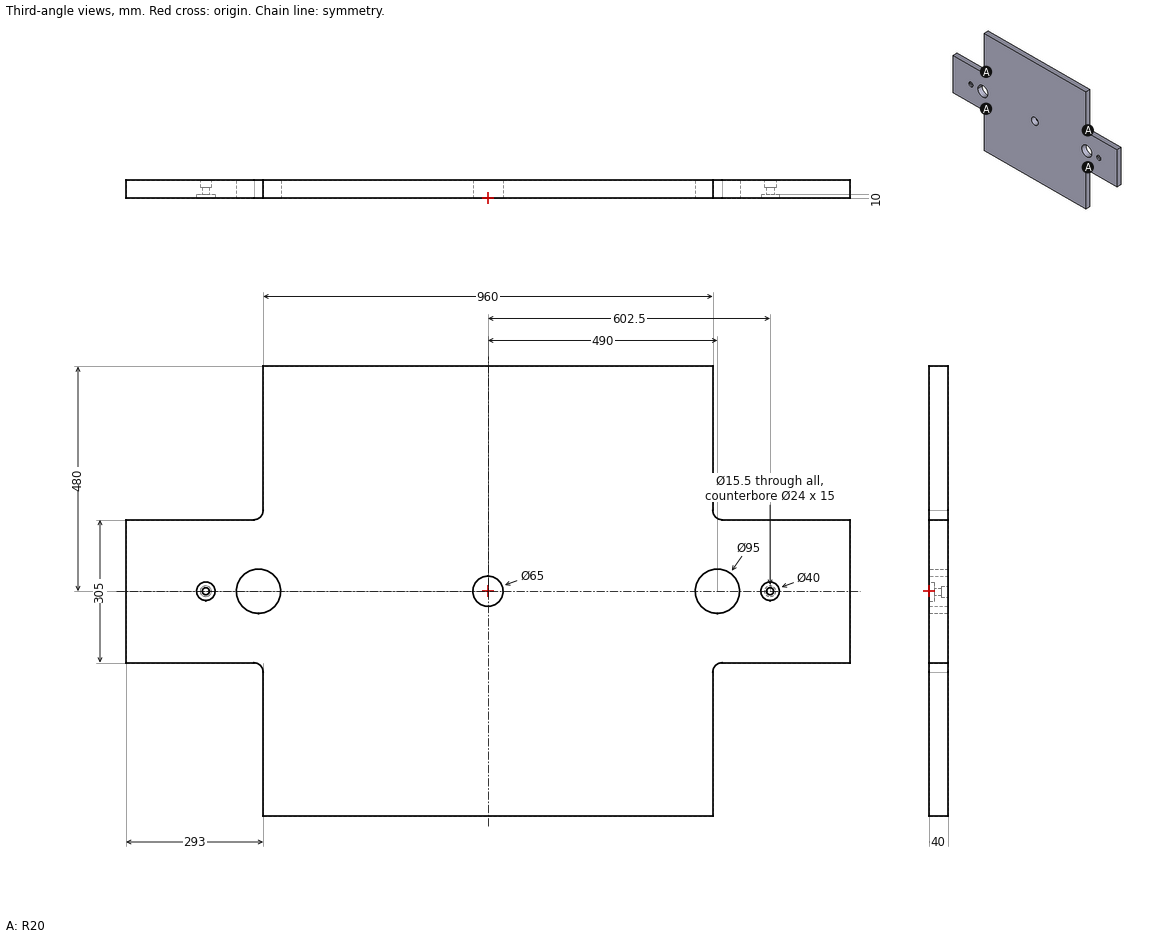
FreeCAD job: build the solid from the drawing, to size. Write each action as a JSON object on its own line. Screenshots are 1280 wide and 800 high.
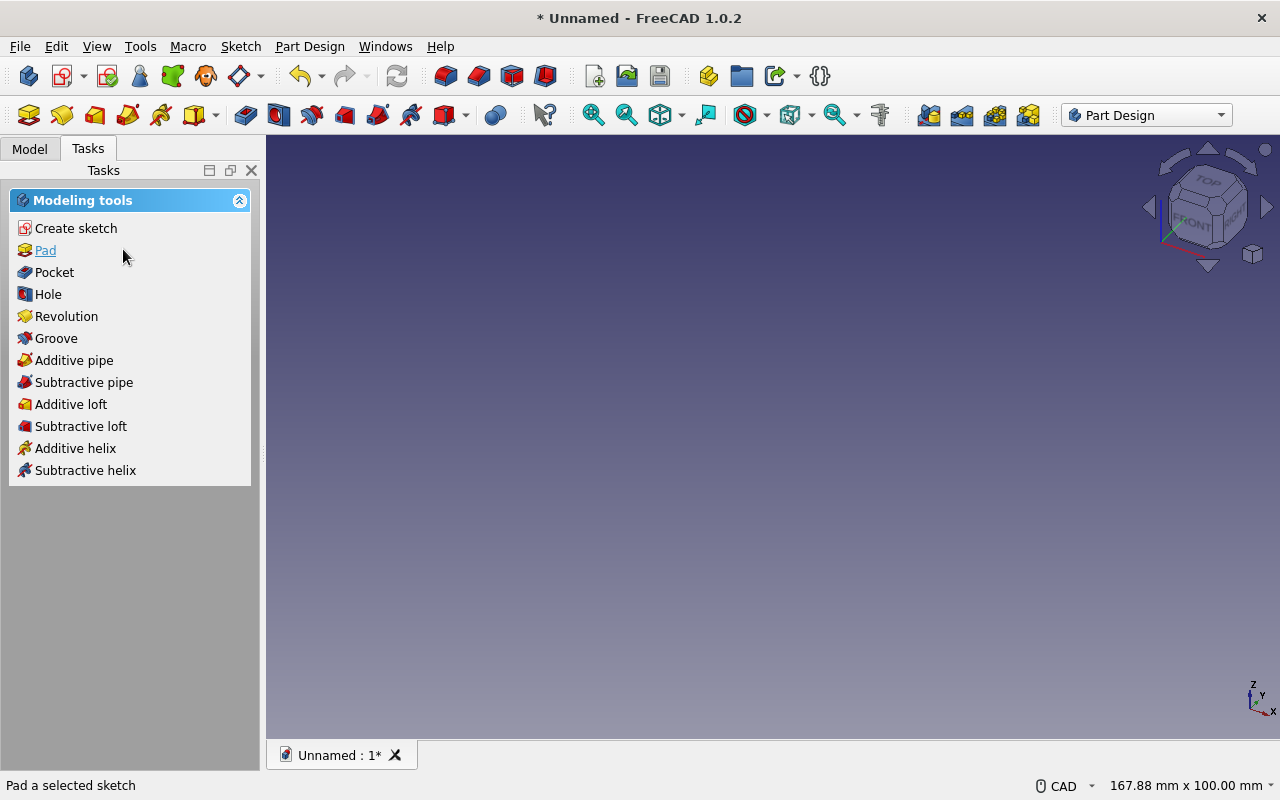
{"action": "left_click", "coordinate": [29, 116]}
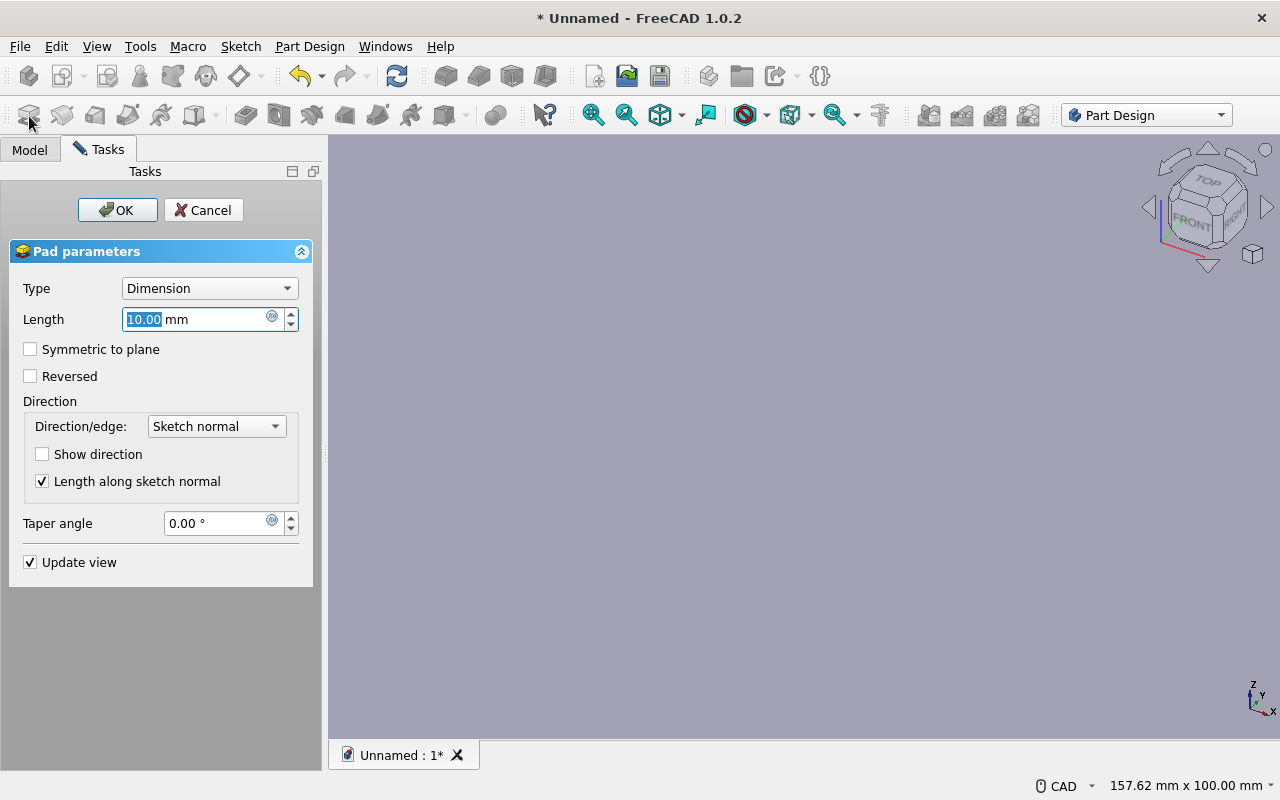
{"action": "type", "text": "40"}
{"action": "key", "text": "Tab"}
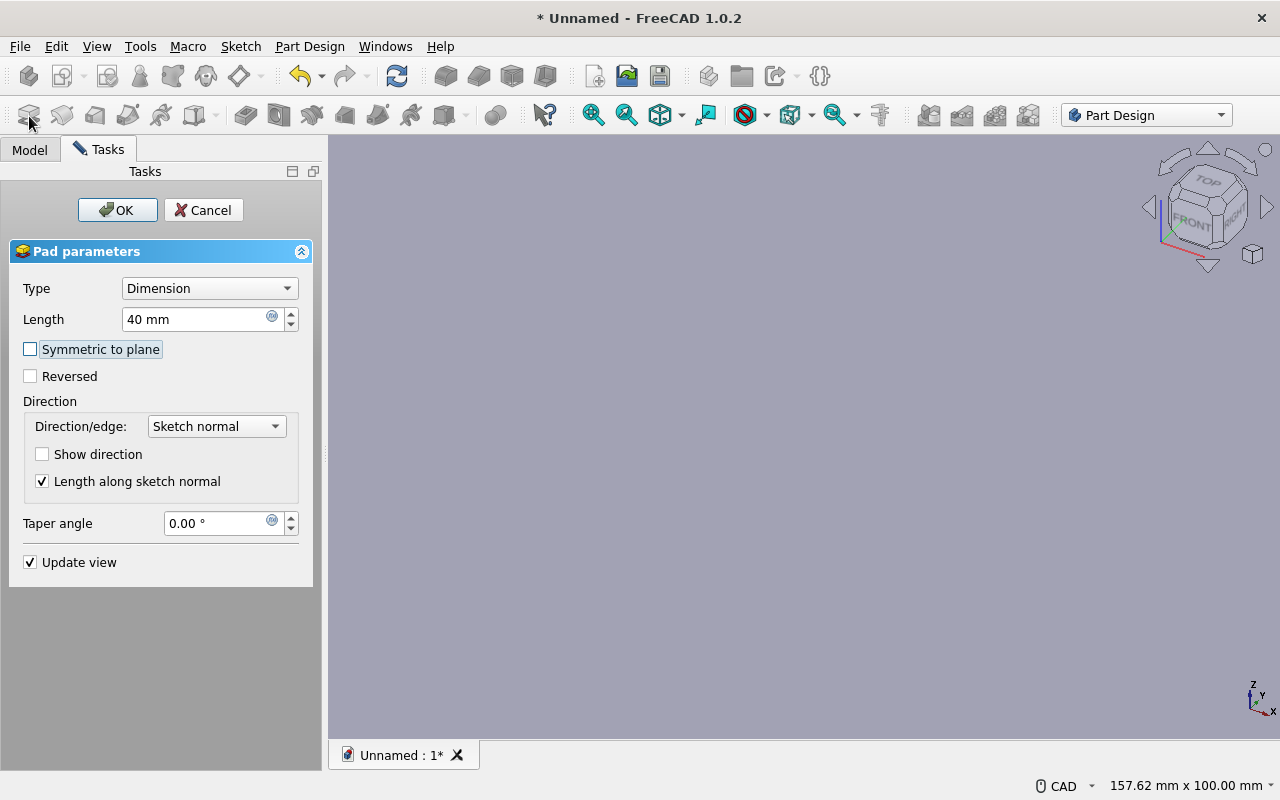
{"action": "left_click", "coordinate": [31, 376]}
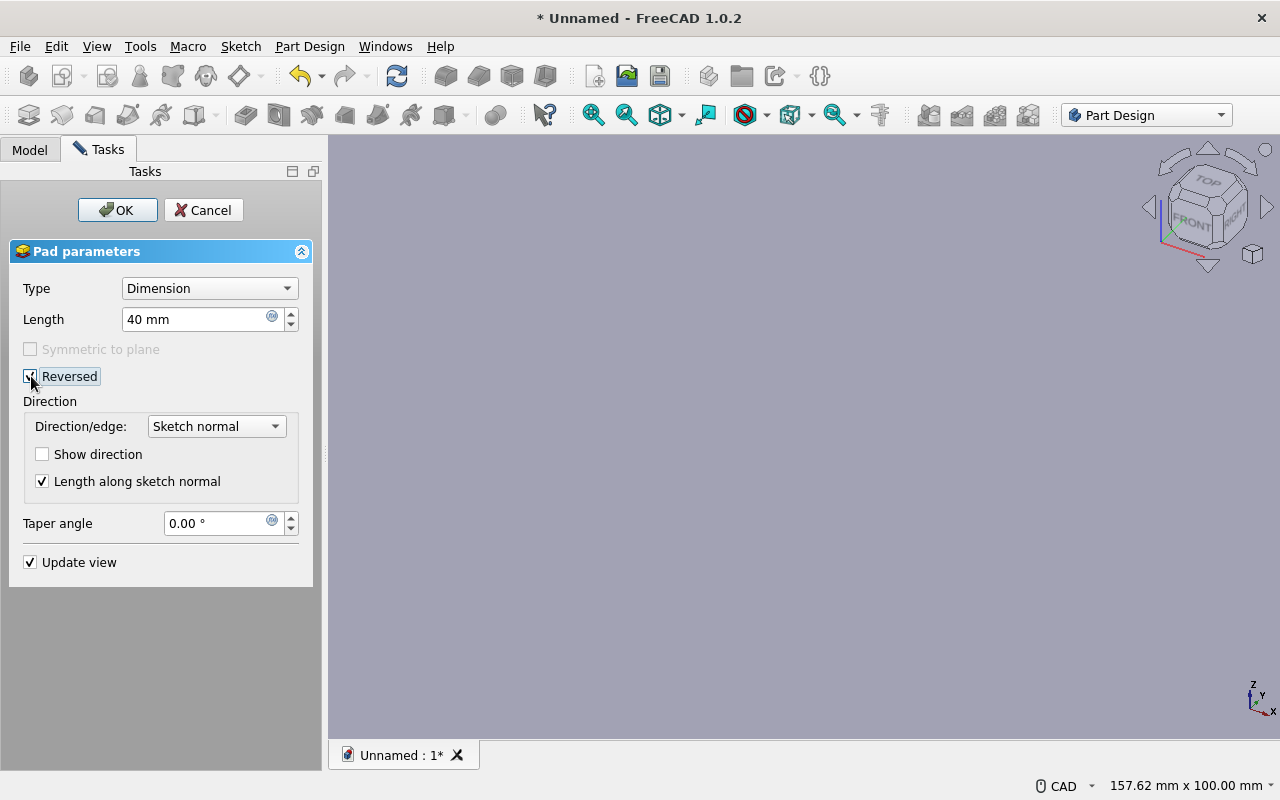
{"action": "left_click", "coordinate": [118, 210]}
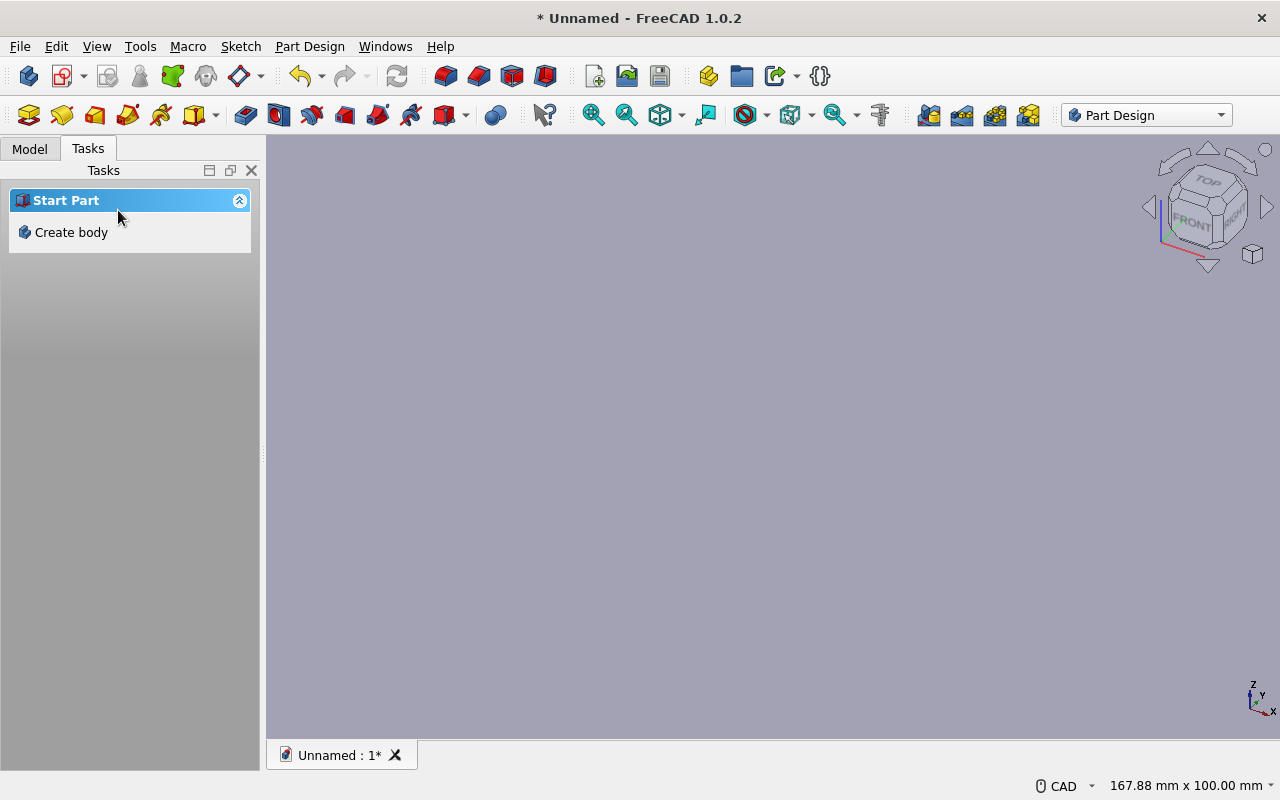
{"action": "key", "text": "v f"}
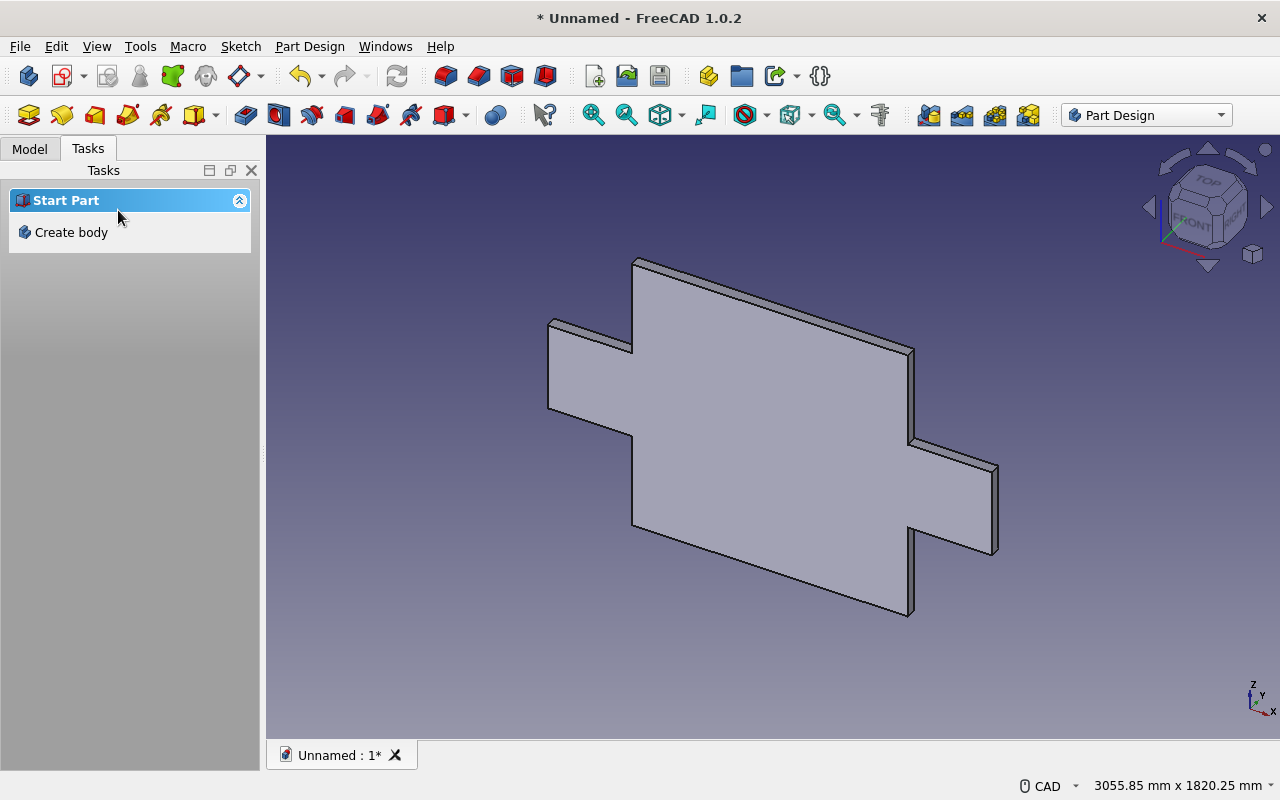
{"action": "left_click", "coordinate": [770, 439]}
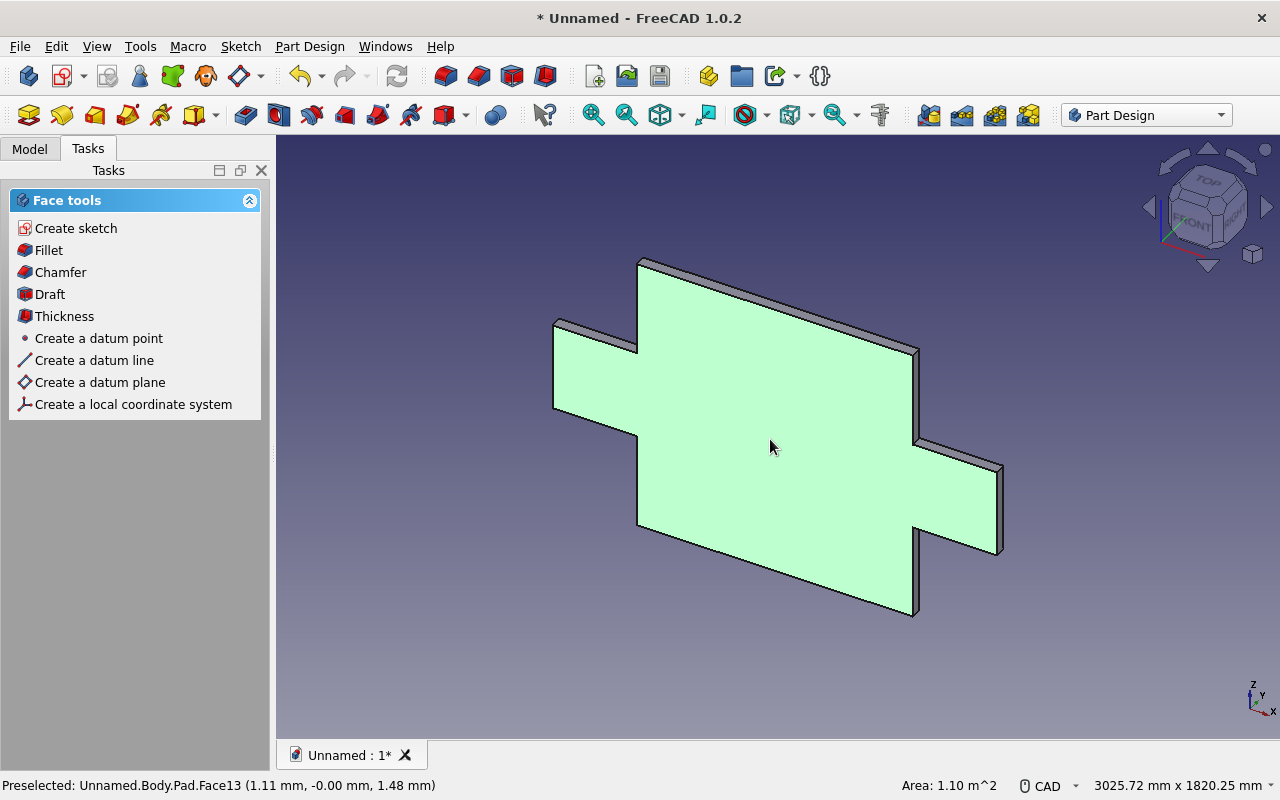
{"action": "left_click", "coordinate": [62, 76]}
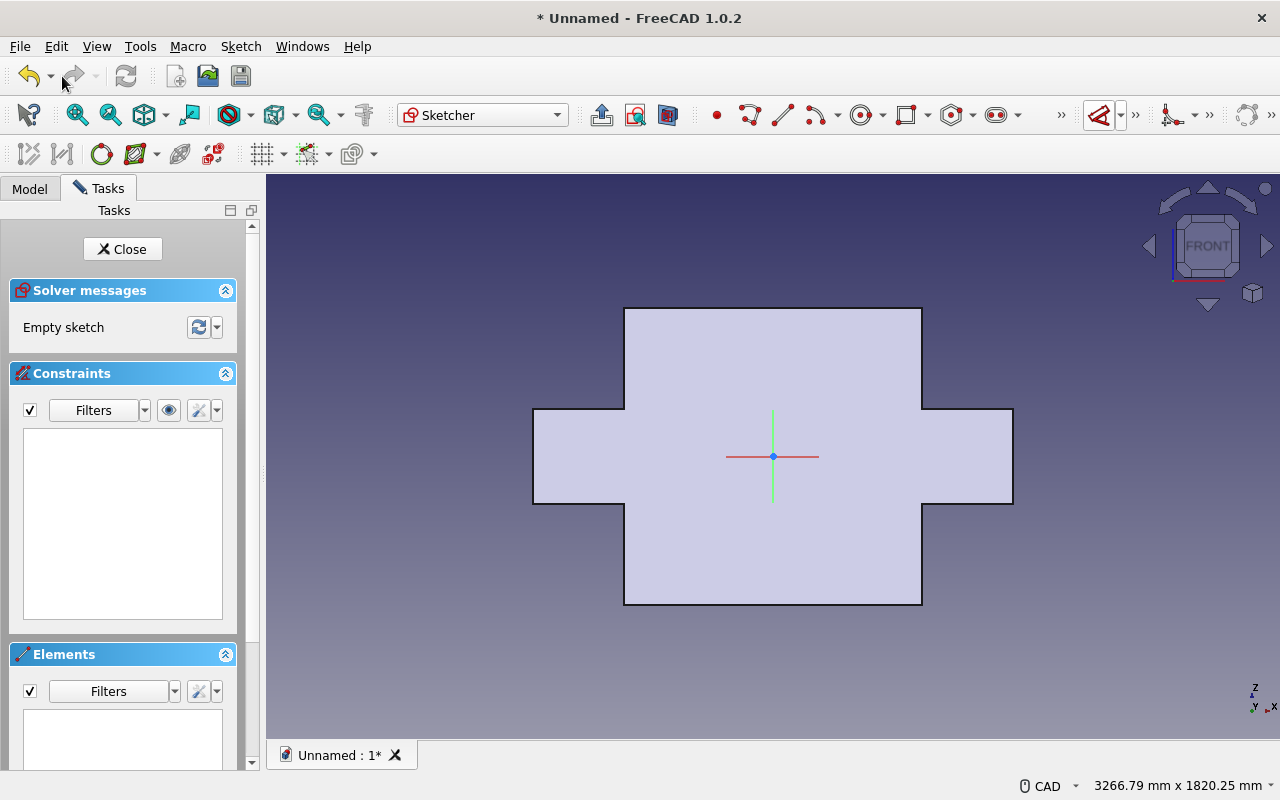
{"action": "scroll", "coordinate": [973, 457], "scroll_direction": "up", "scroll_amount": 15}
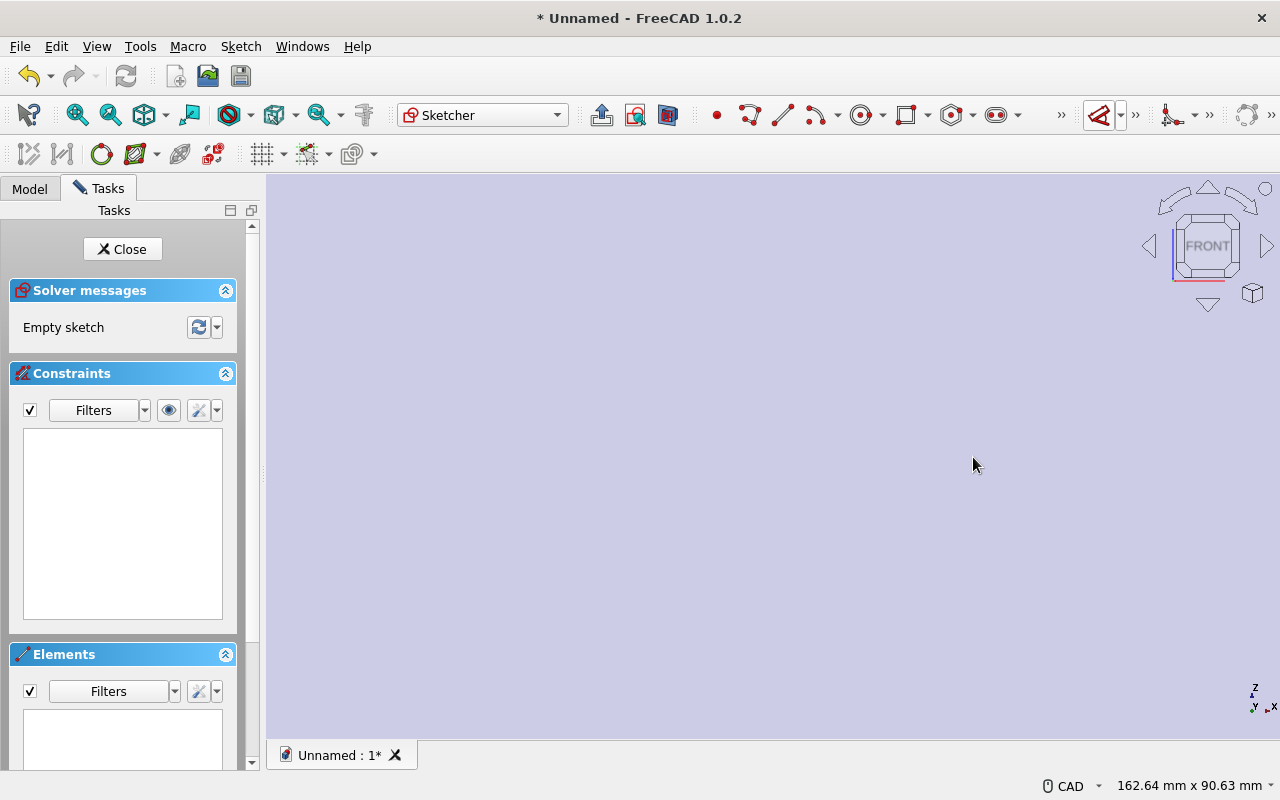
{"action": "scroll", "coordinate": [687, 399], "scroll_direction": "up", "scroll_amount": 2}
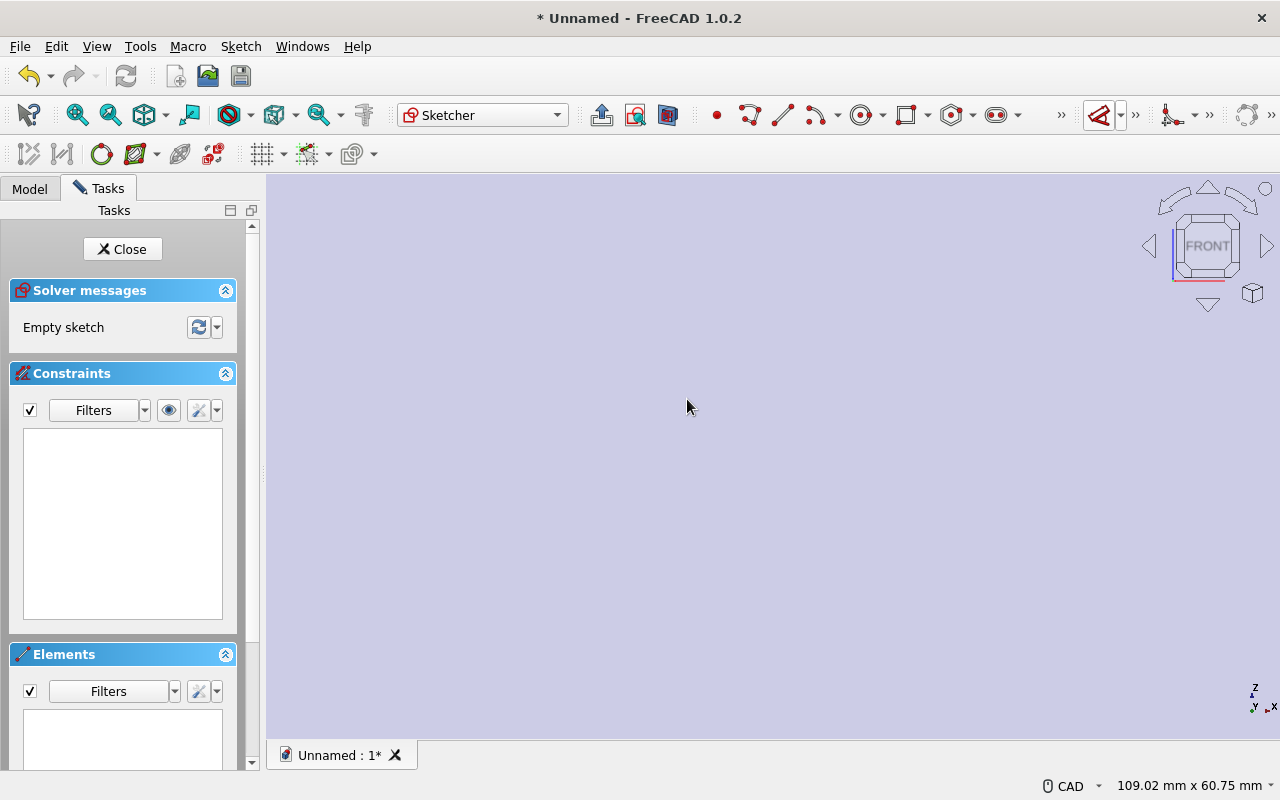
{"action": "key", "text": "g c"}